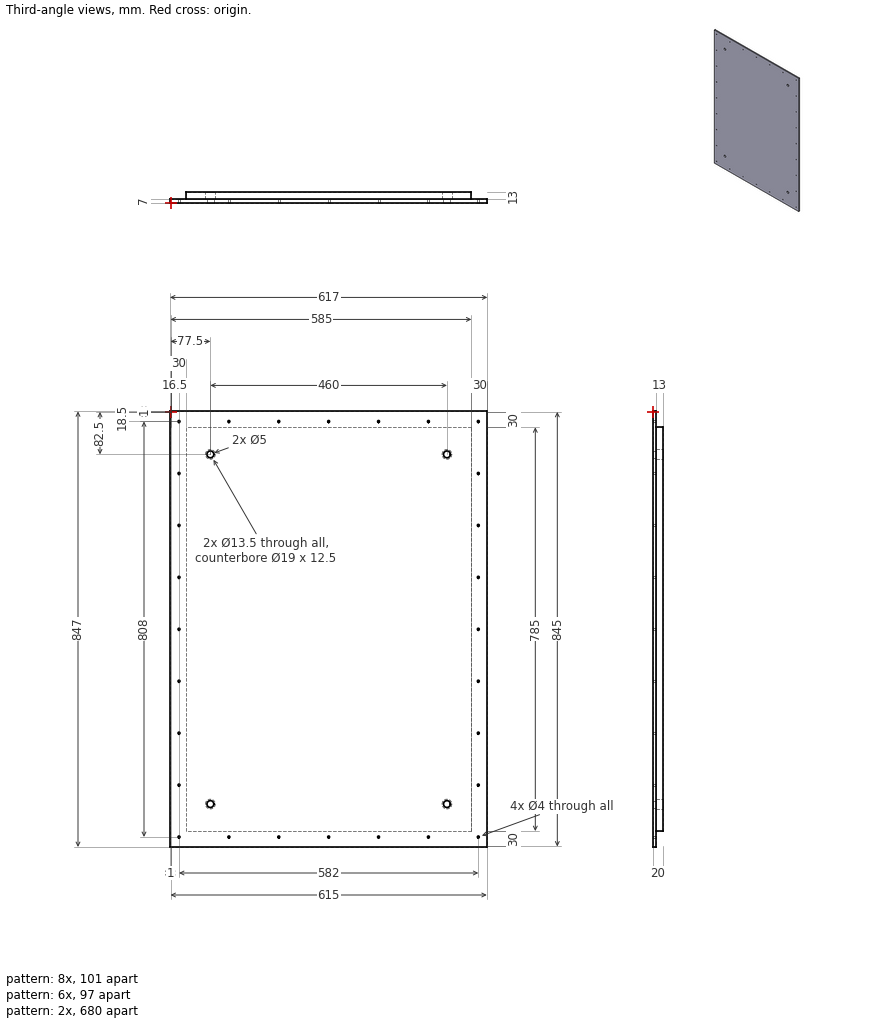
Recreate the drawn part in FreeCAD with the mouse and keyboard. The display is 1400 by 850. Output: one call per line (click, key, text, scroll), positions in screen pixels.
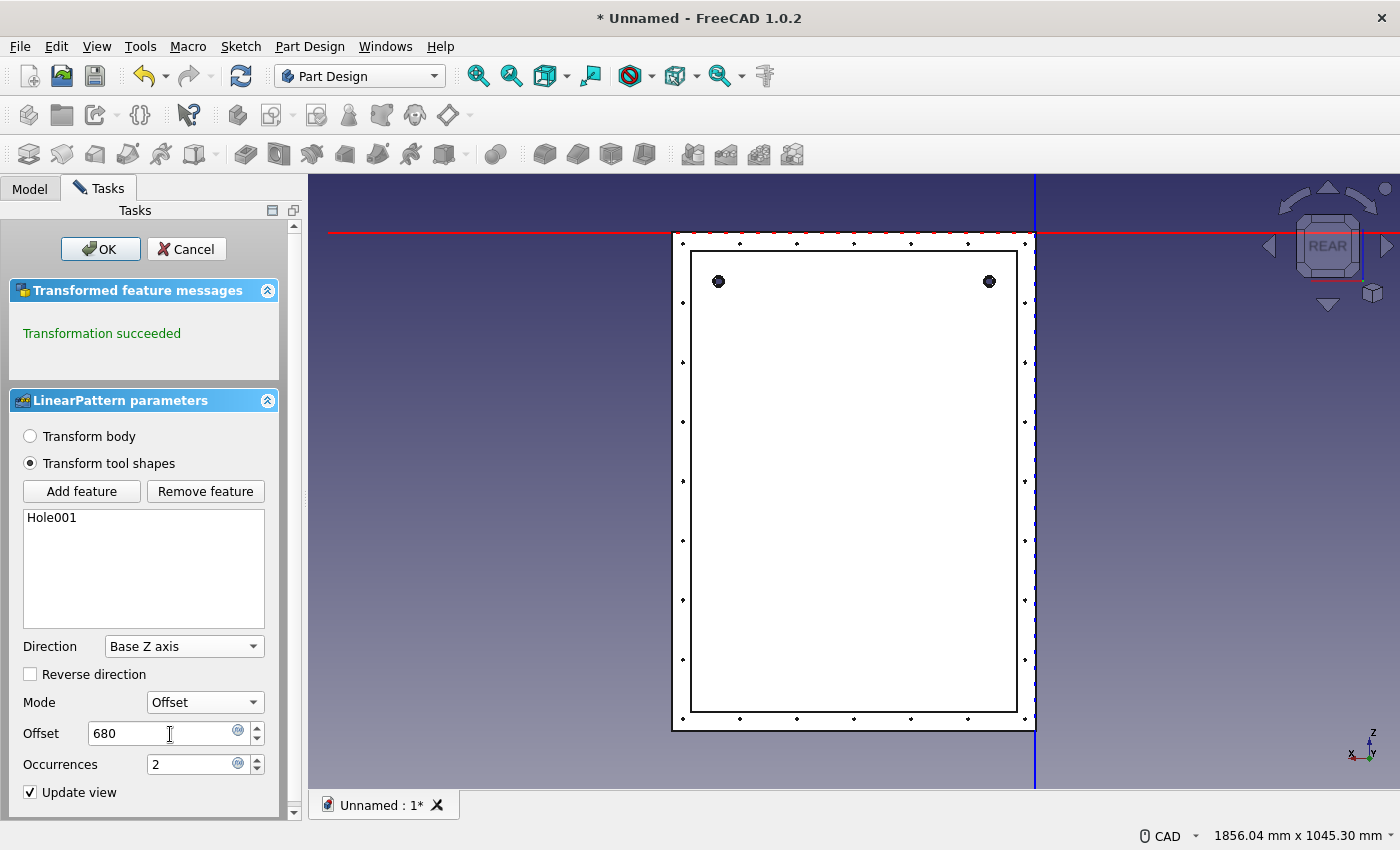
triple_click(199, 764)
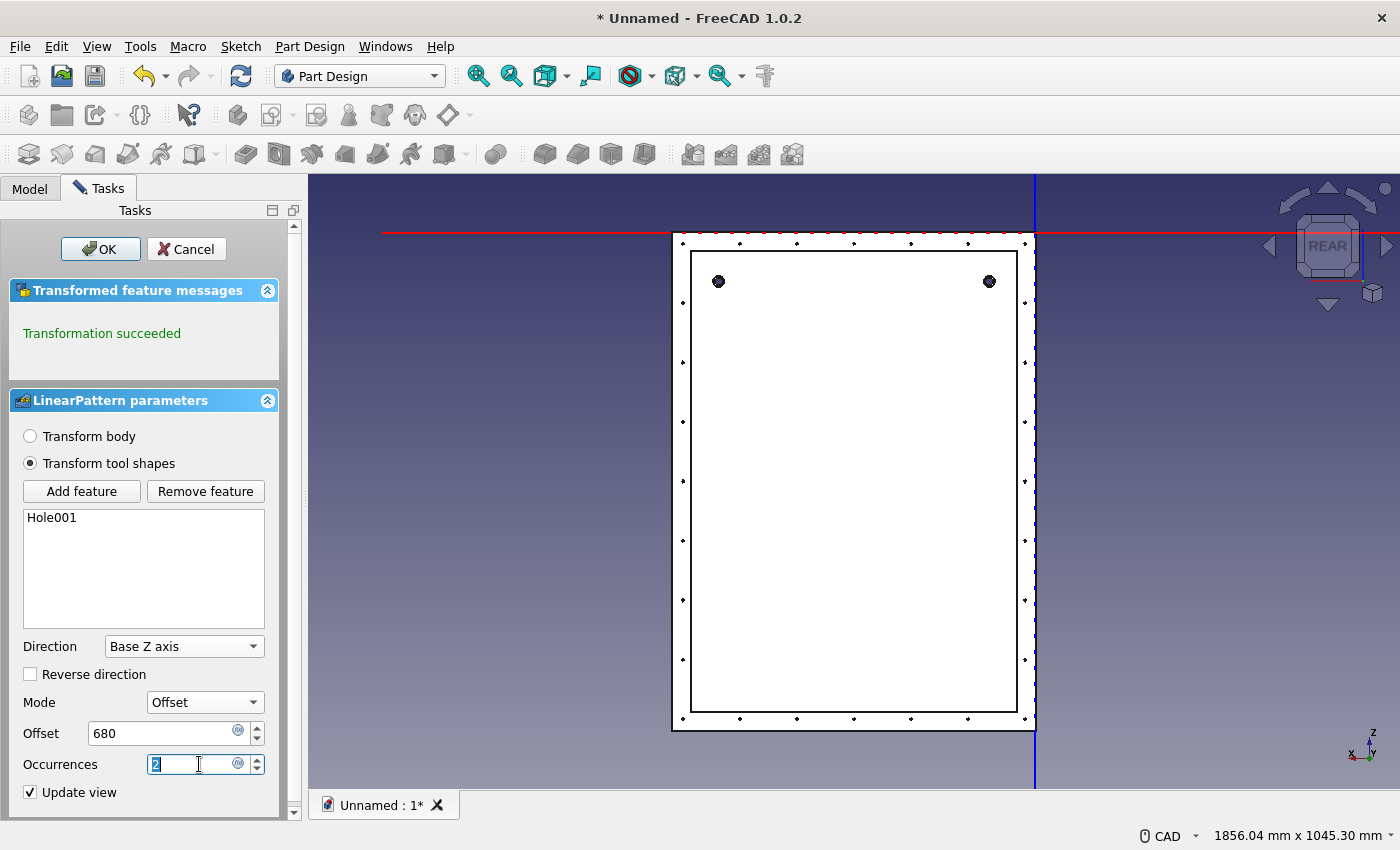
text(2)
key(Tab)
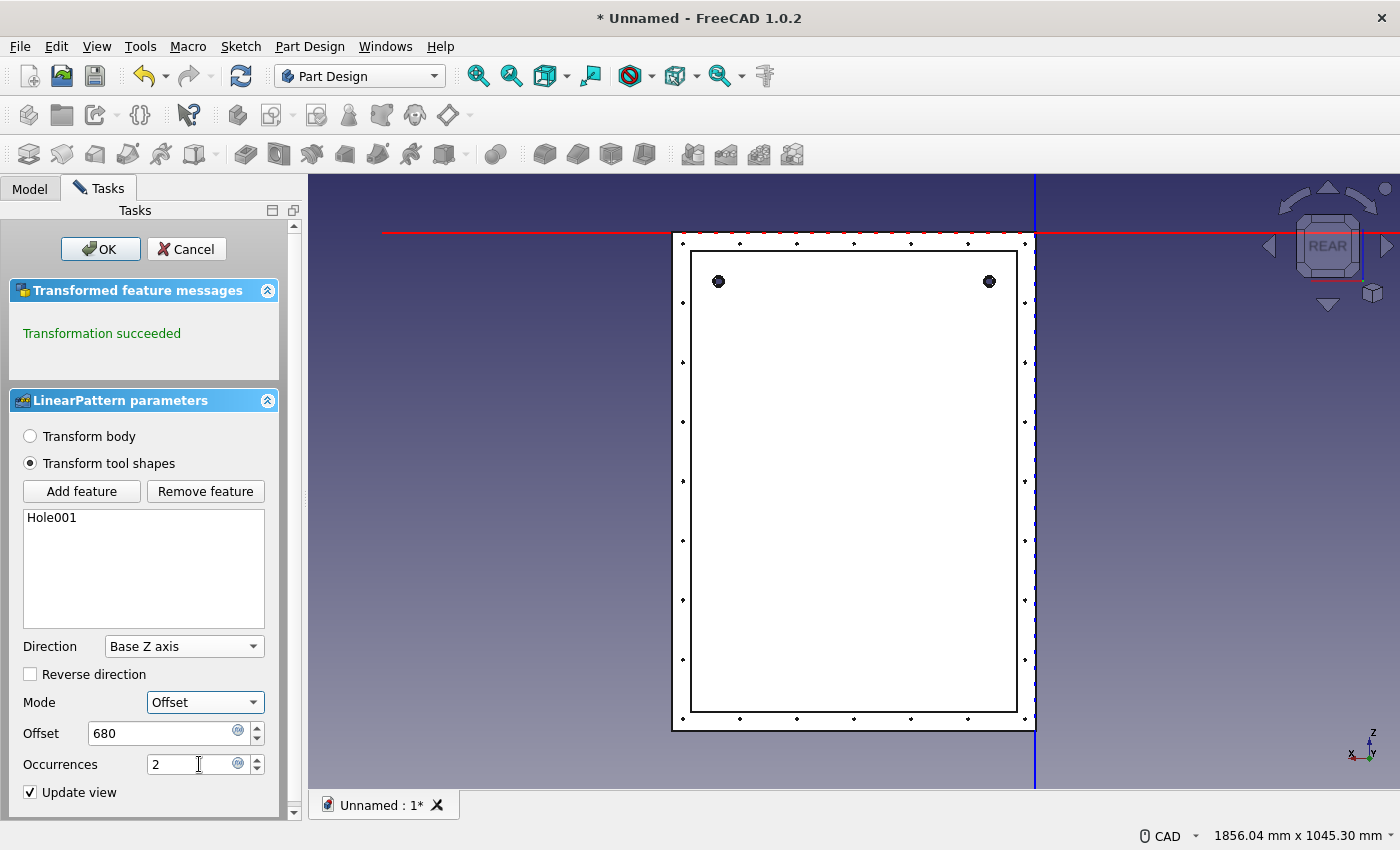
click(31, 674)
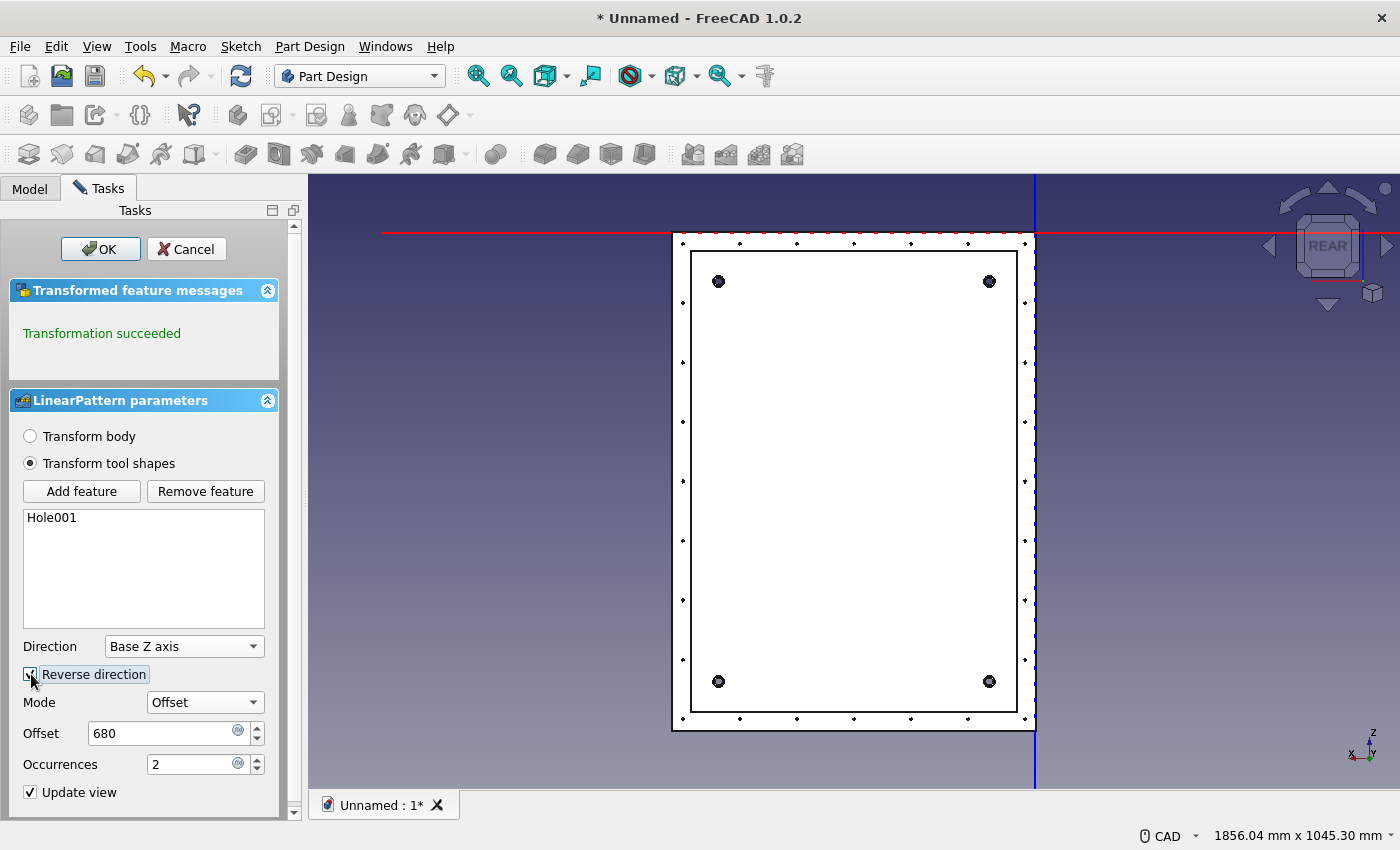
click(101, 249)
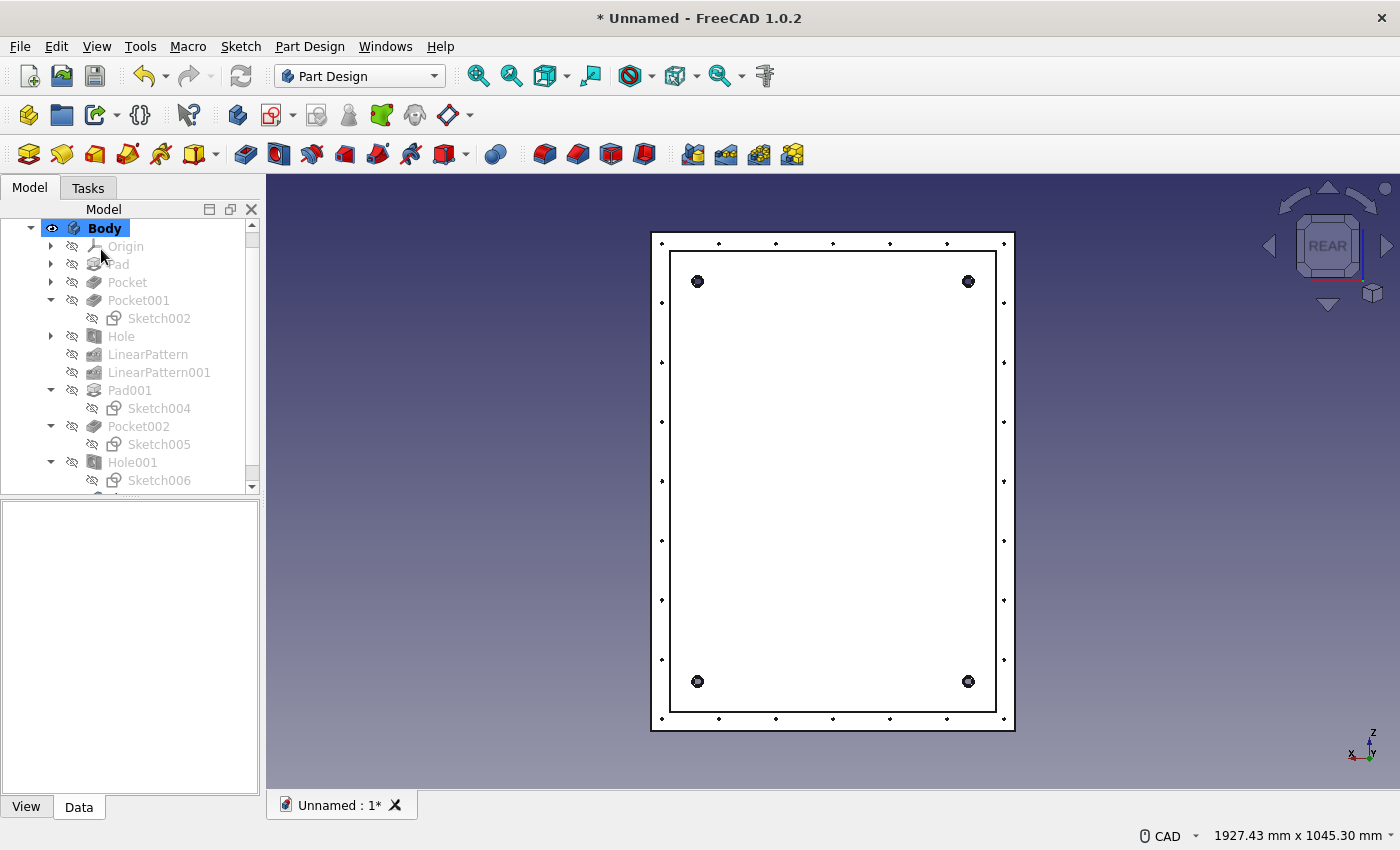
key(0)